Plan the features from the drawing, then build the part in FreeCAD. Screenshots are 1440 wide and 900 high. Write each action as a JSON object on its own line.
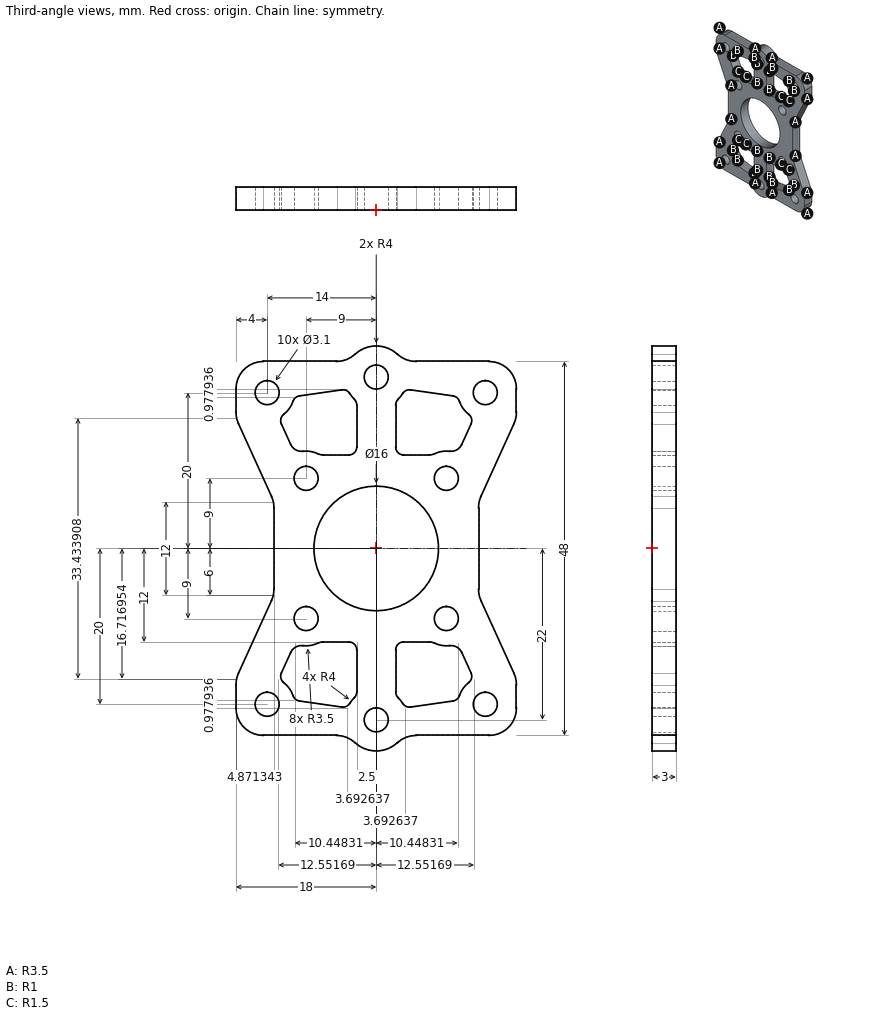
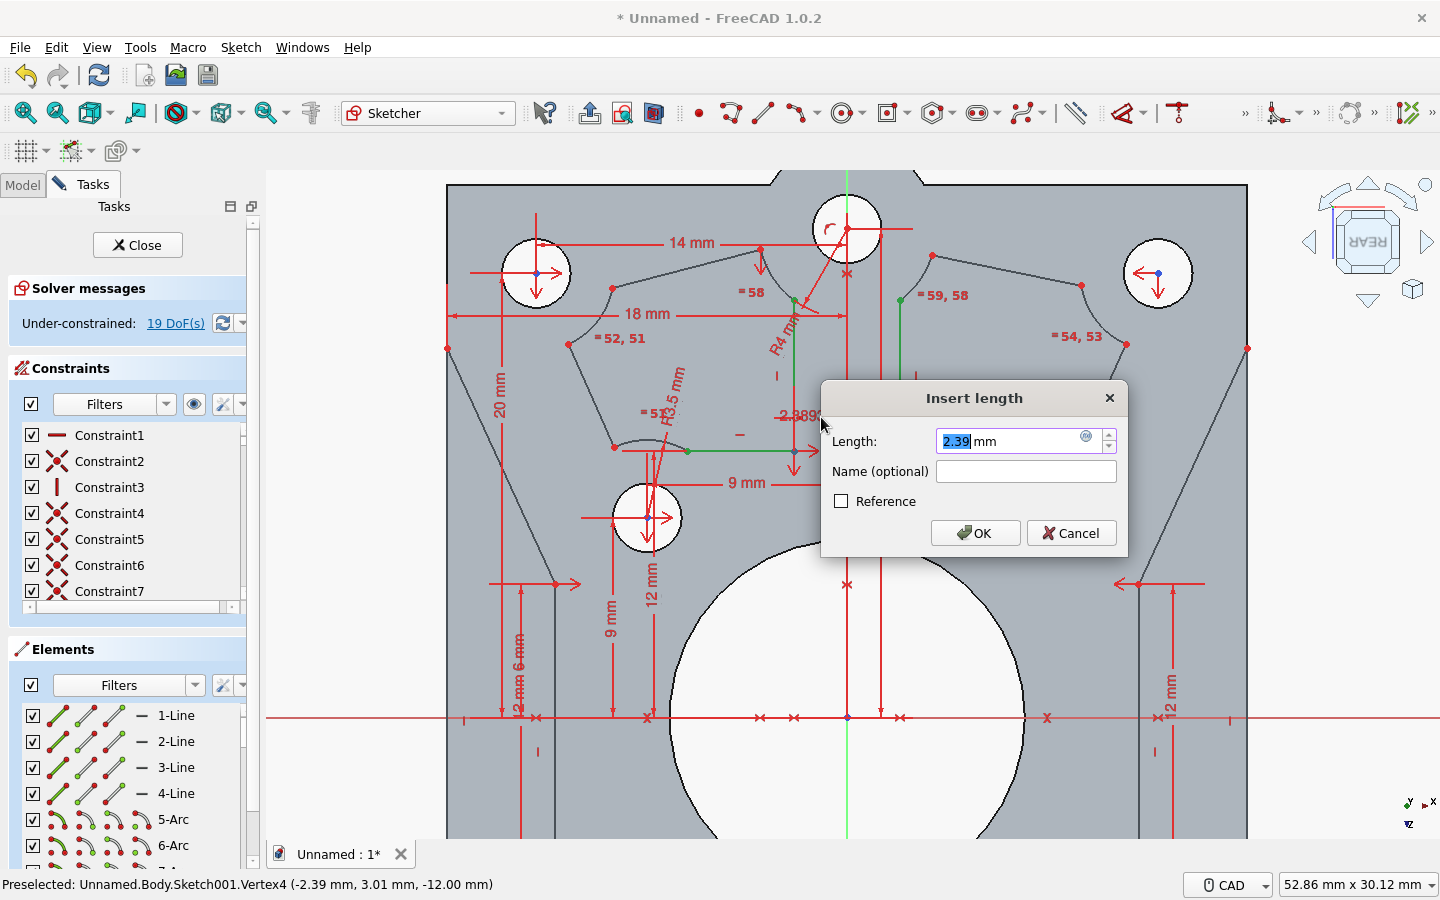
{"action": "type", "text": "2.5"}
{"action": "key", "text": "Return"}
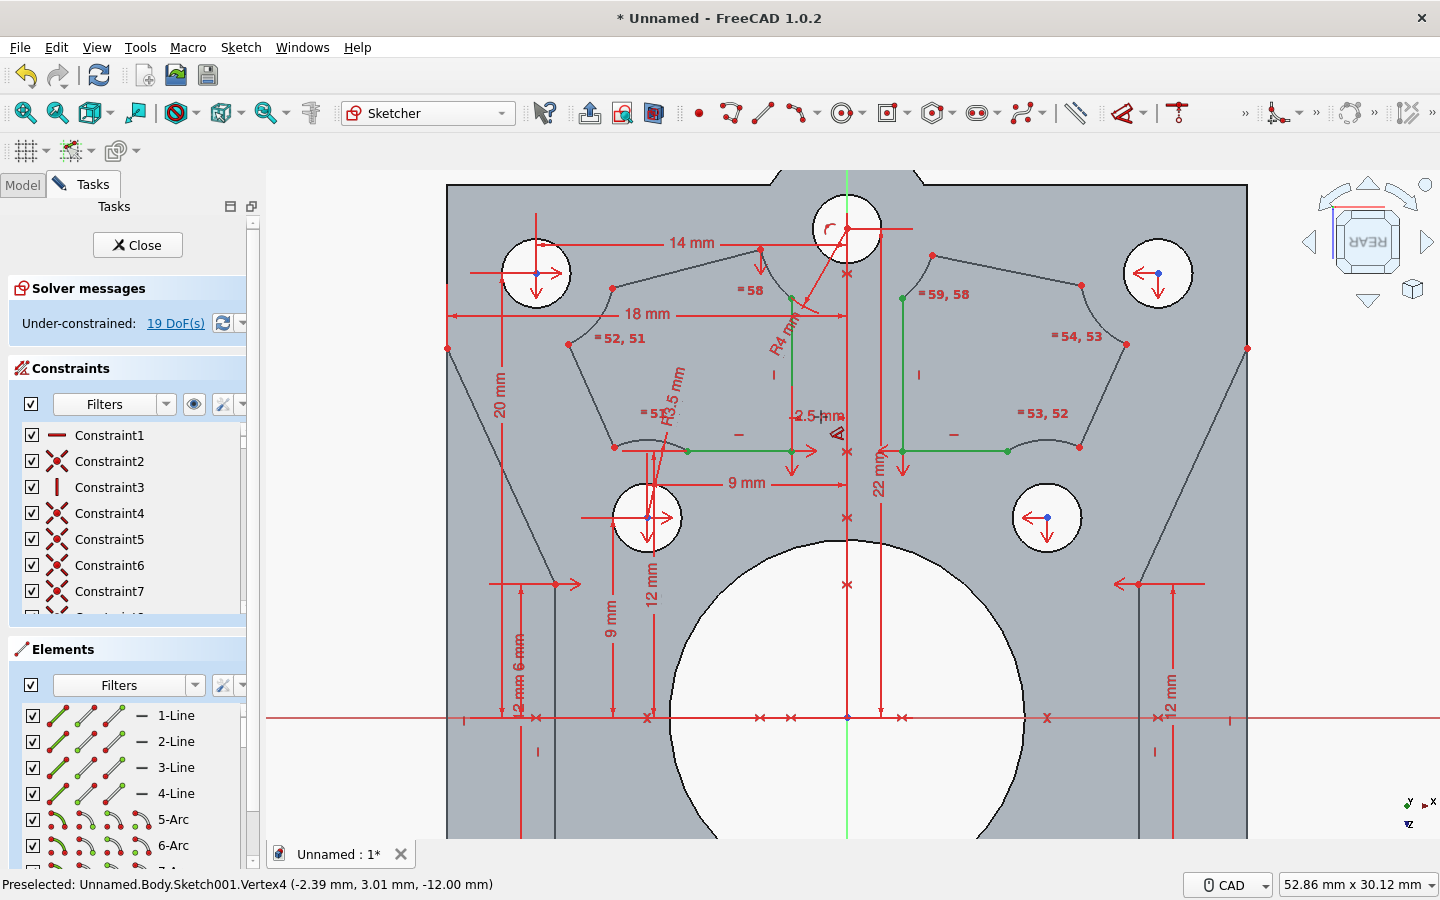
{"action": "left_click", "coordinate": [447, 572]}
{"action": "left_click", "coordinate": [413, 580]}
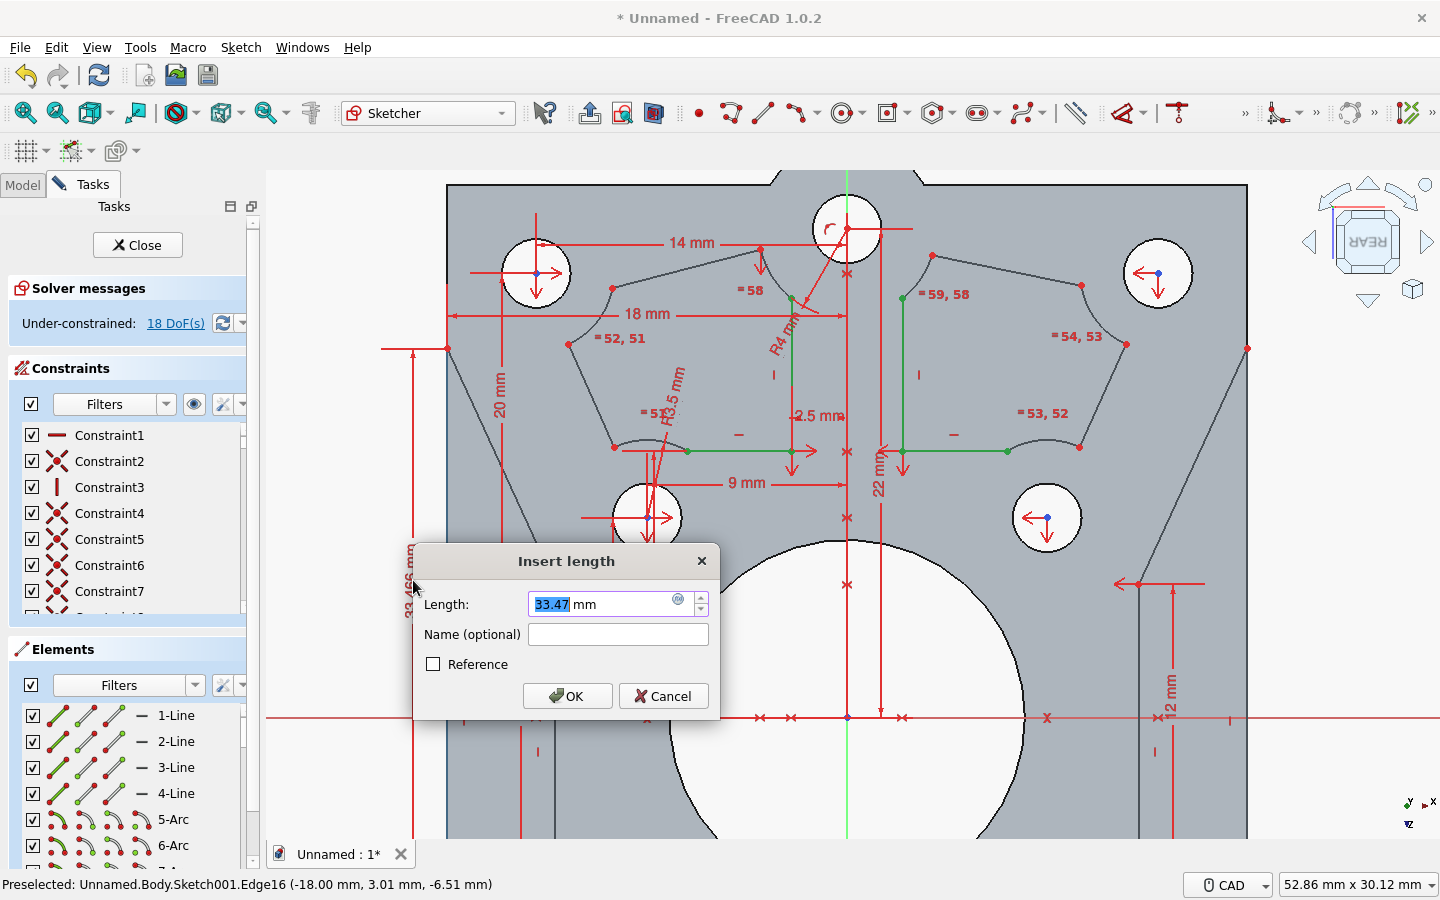
{"action": "type", "text": "33.433908"}
{"action": "key", "text": "Return"}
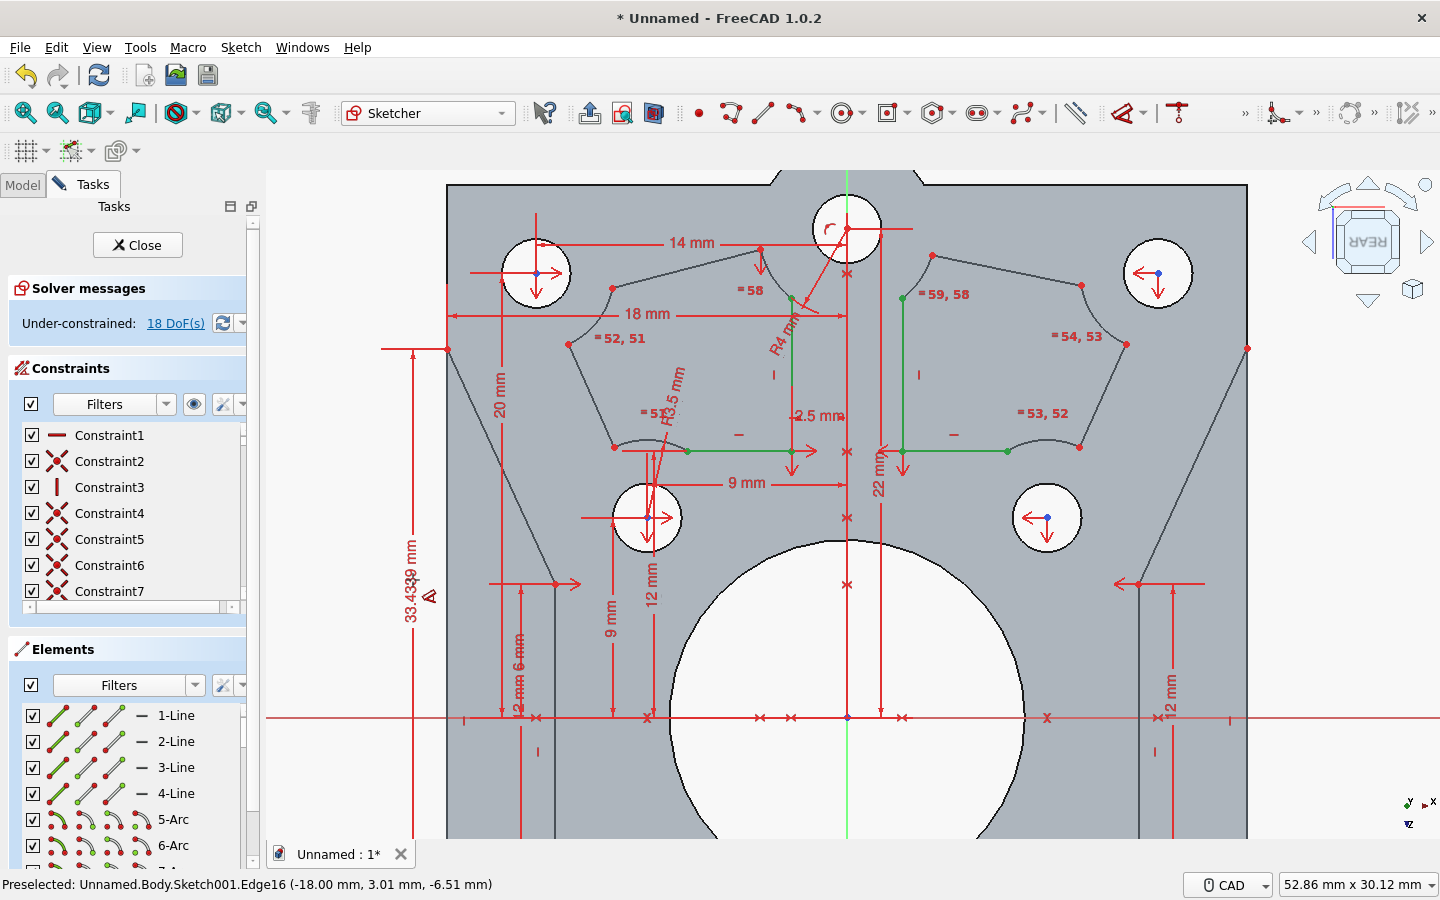
{"action": "left_click", "coordinate": [1247, 572]}
{"action": "left_click", "coordinate": [1213, 580]}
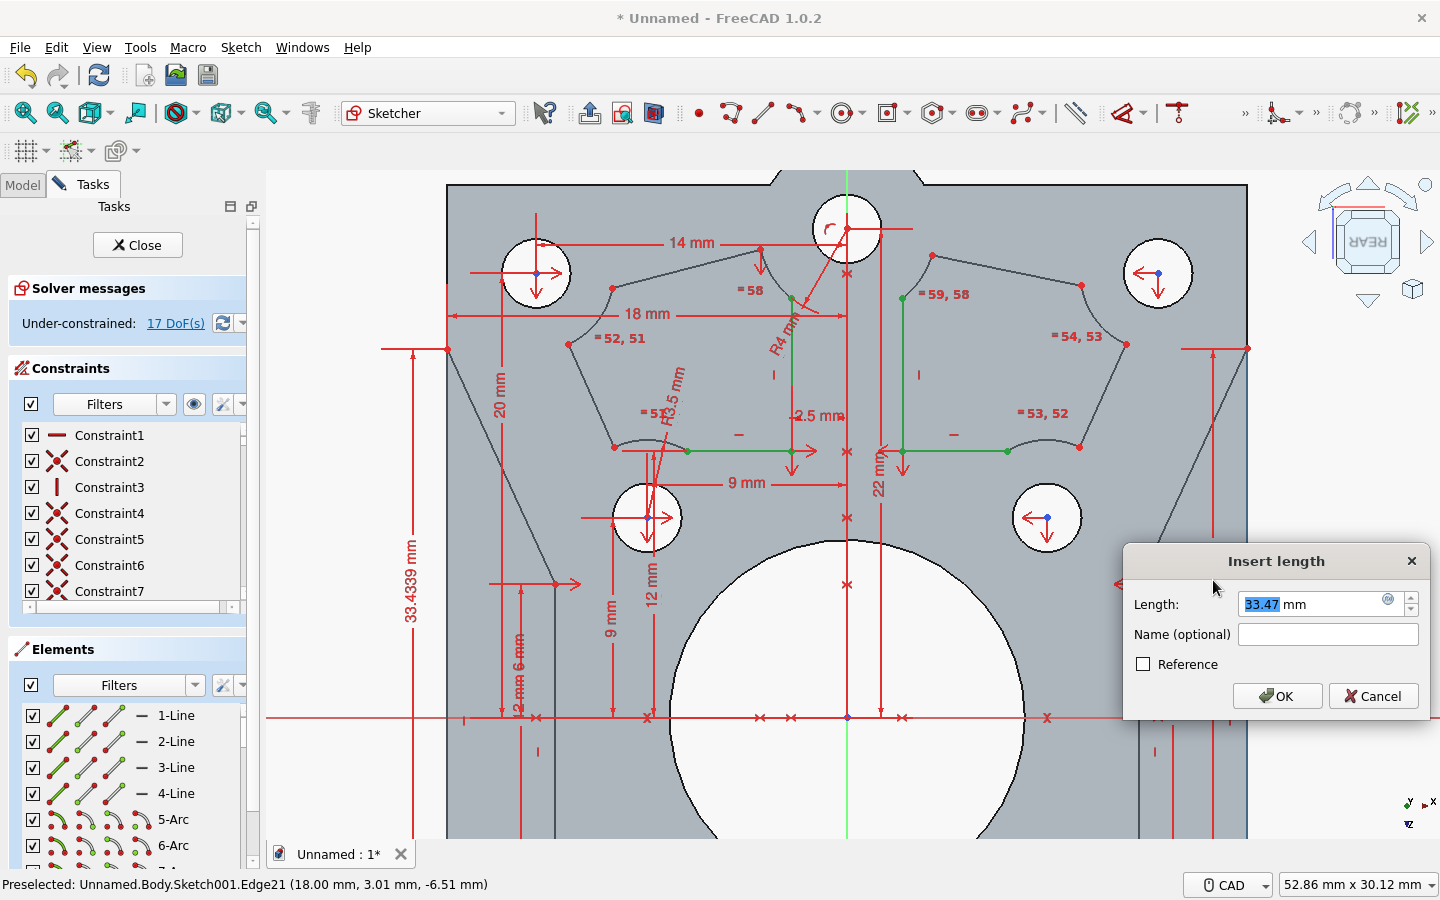
{"action": "type", "text": "33.433908"}
{"action": "key", "text": "Return"}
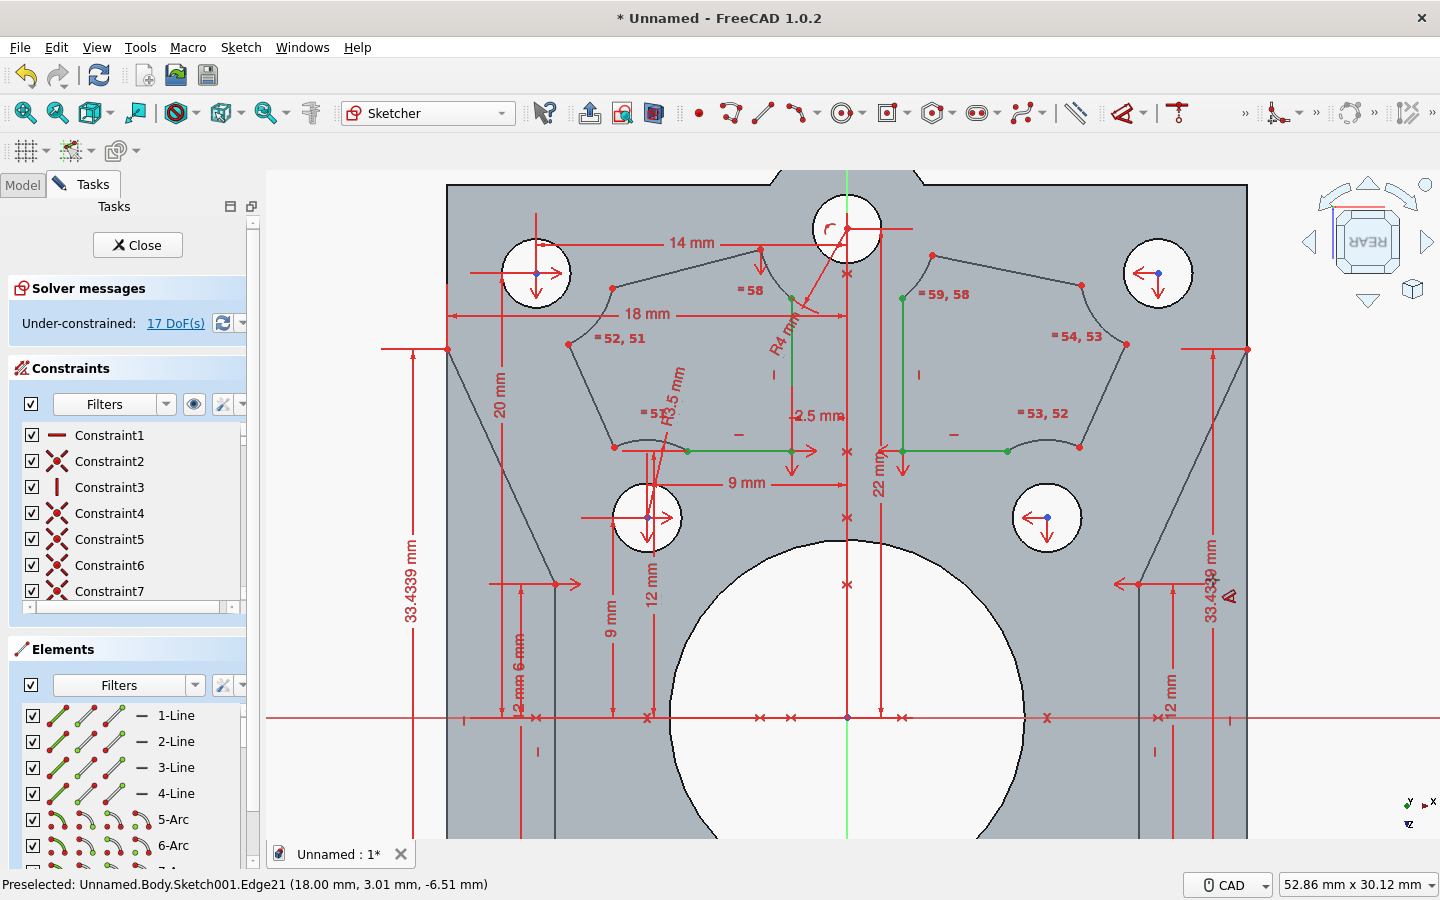
{"action": "left_click", "coordinate": [568, 344]}
{"action": "left_click", "coordinate": [772, 310]}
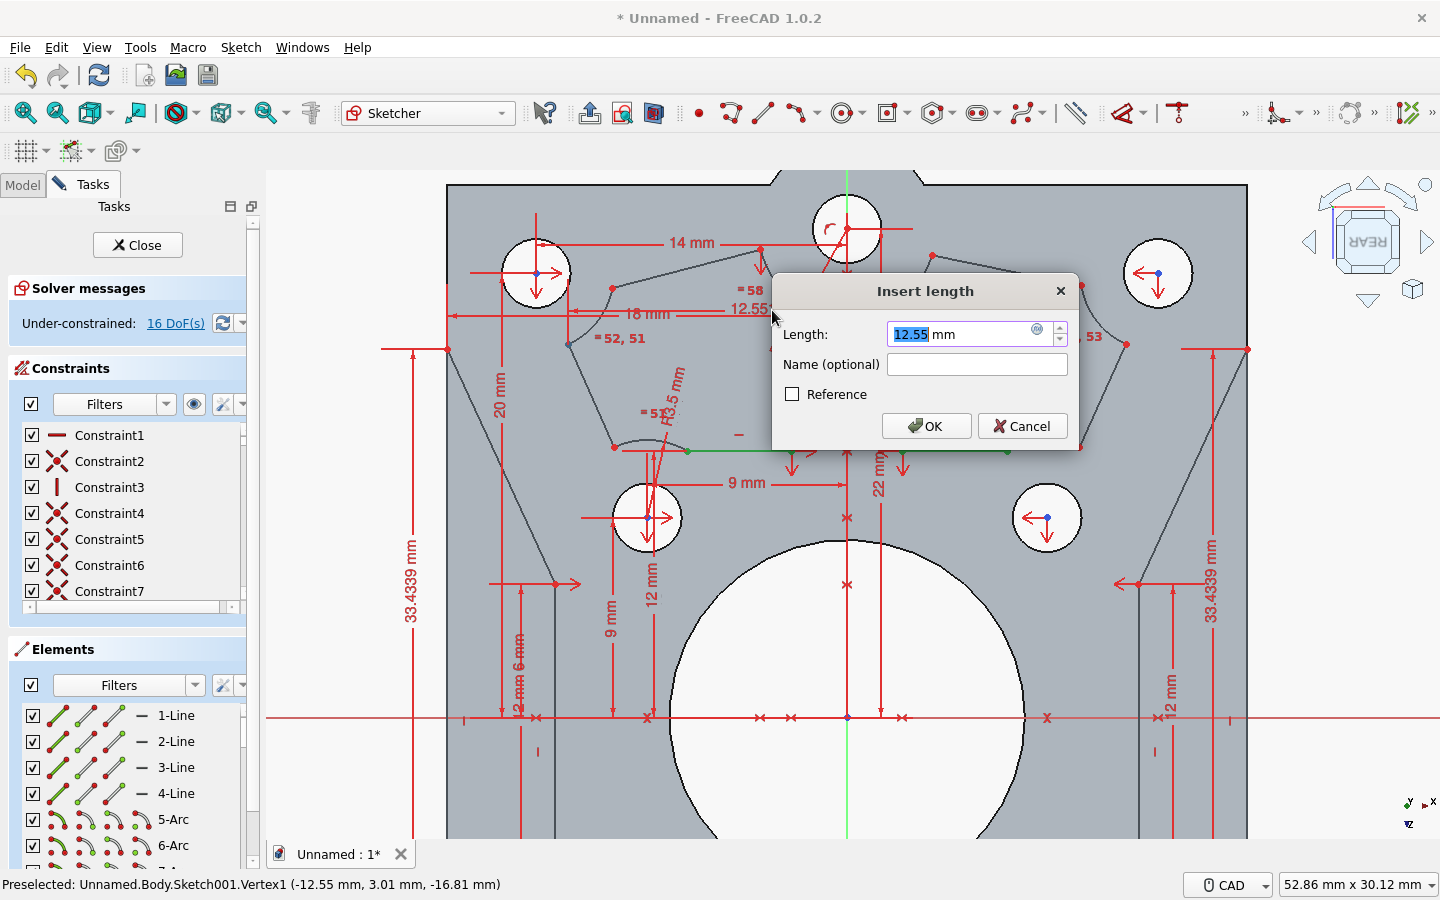
{"action": "type", "text": "12.55169"}
{"action": "key", "text": "Return"}